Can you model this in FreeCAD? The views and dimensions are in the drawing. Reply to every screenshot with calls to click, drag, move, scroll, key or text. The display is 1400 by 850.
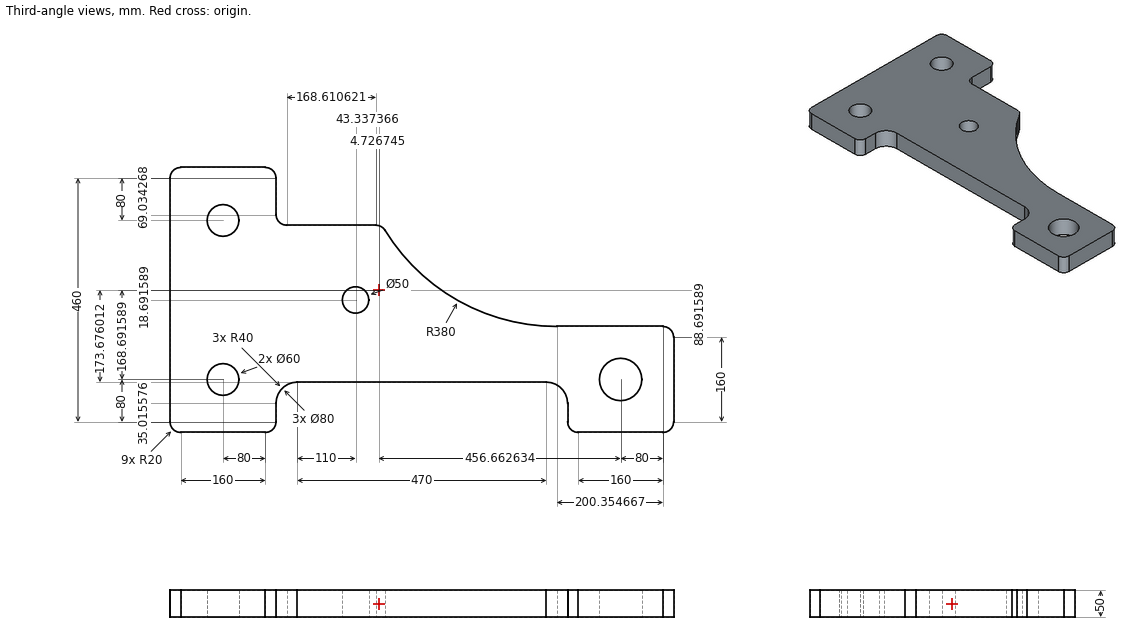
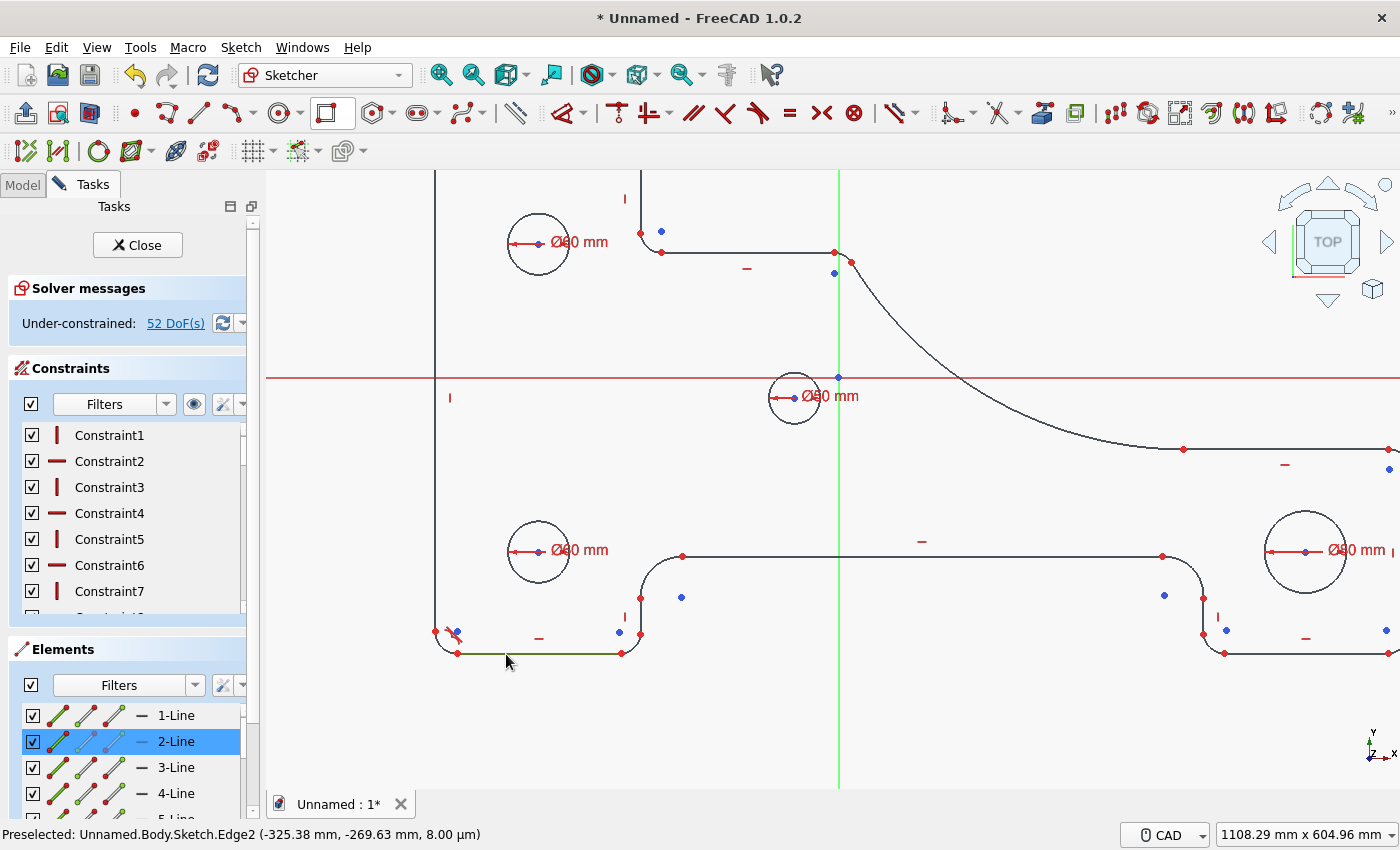
click(634, 648)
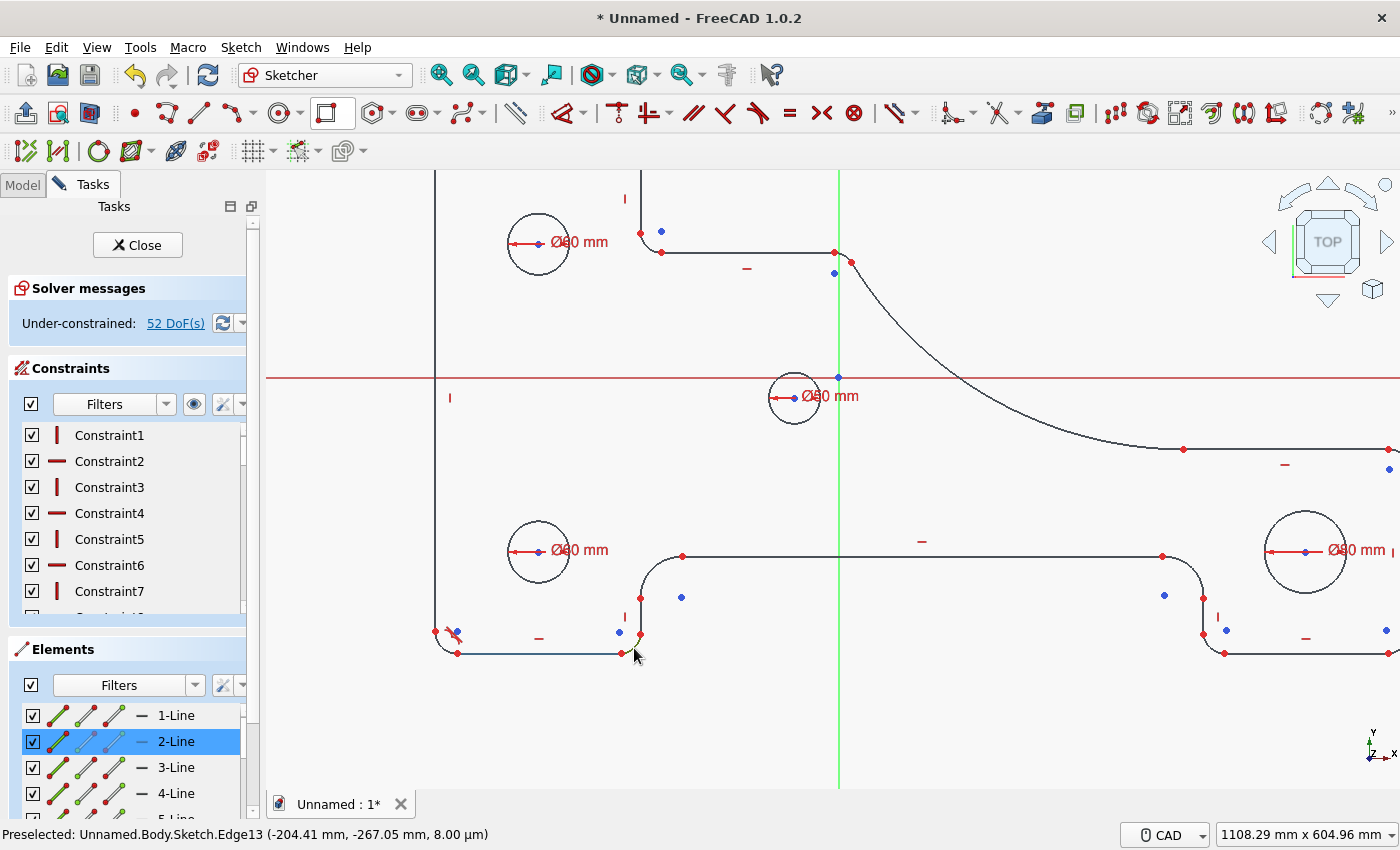
click(758, 114)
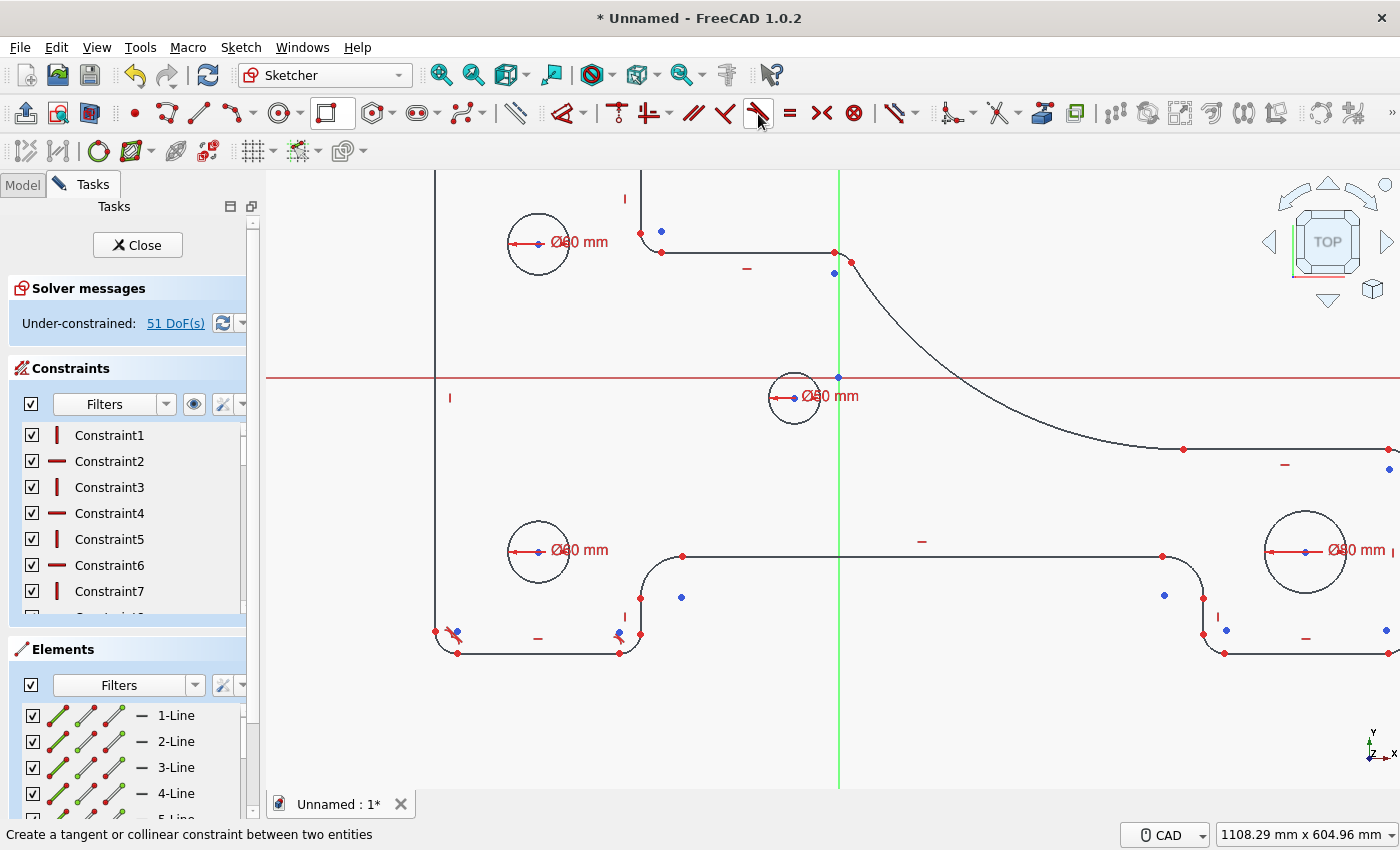
scroll(641, 624, up, 2)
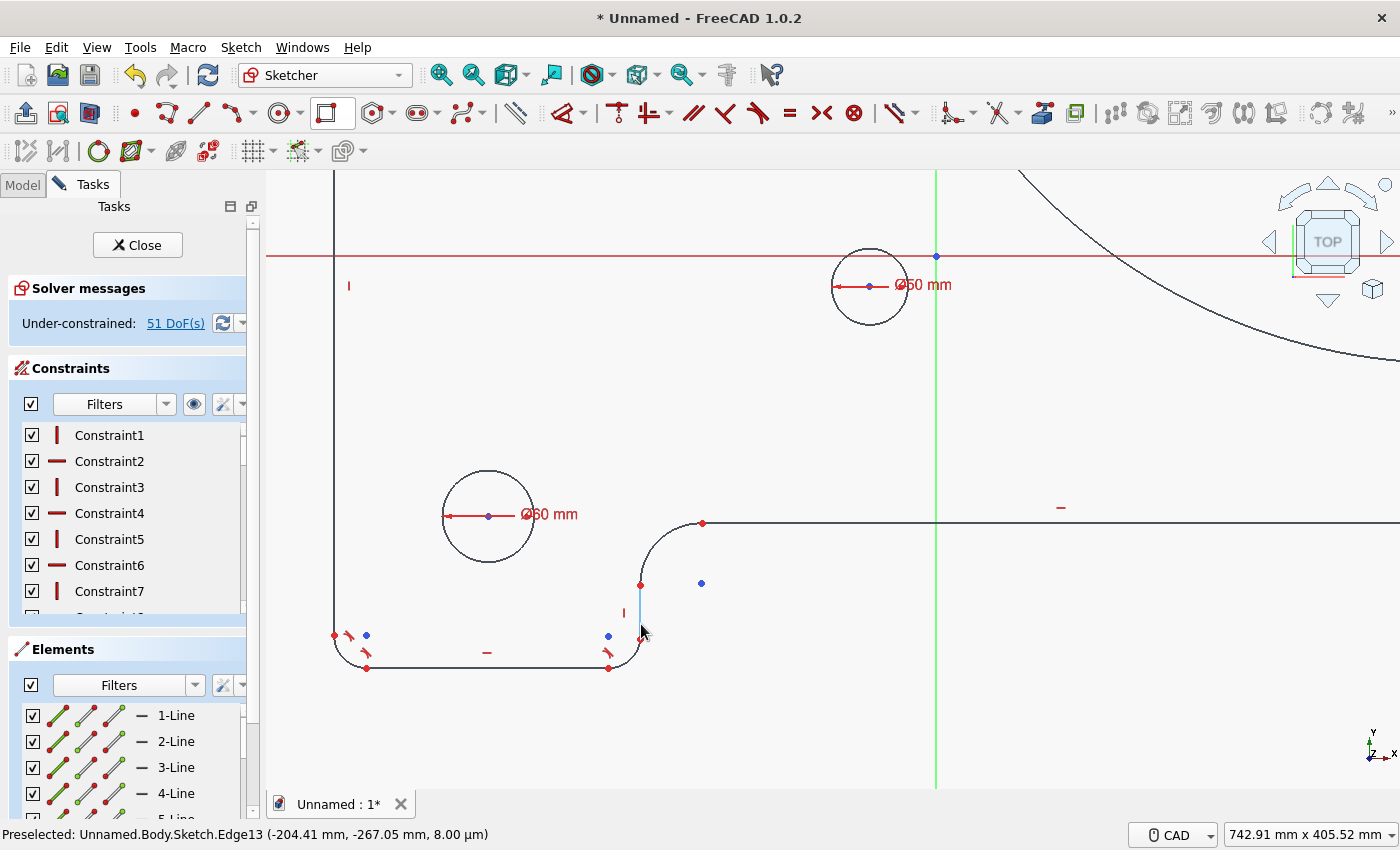
click(640, 623)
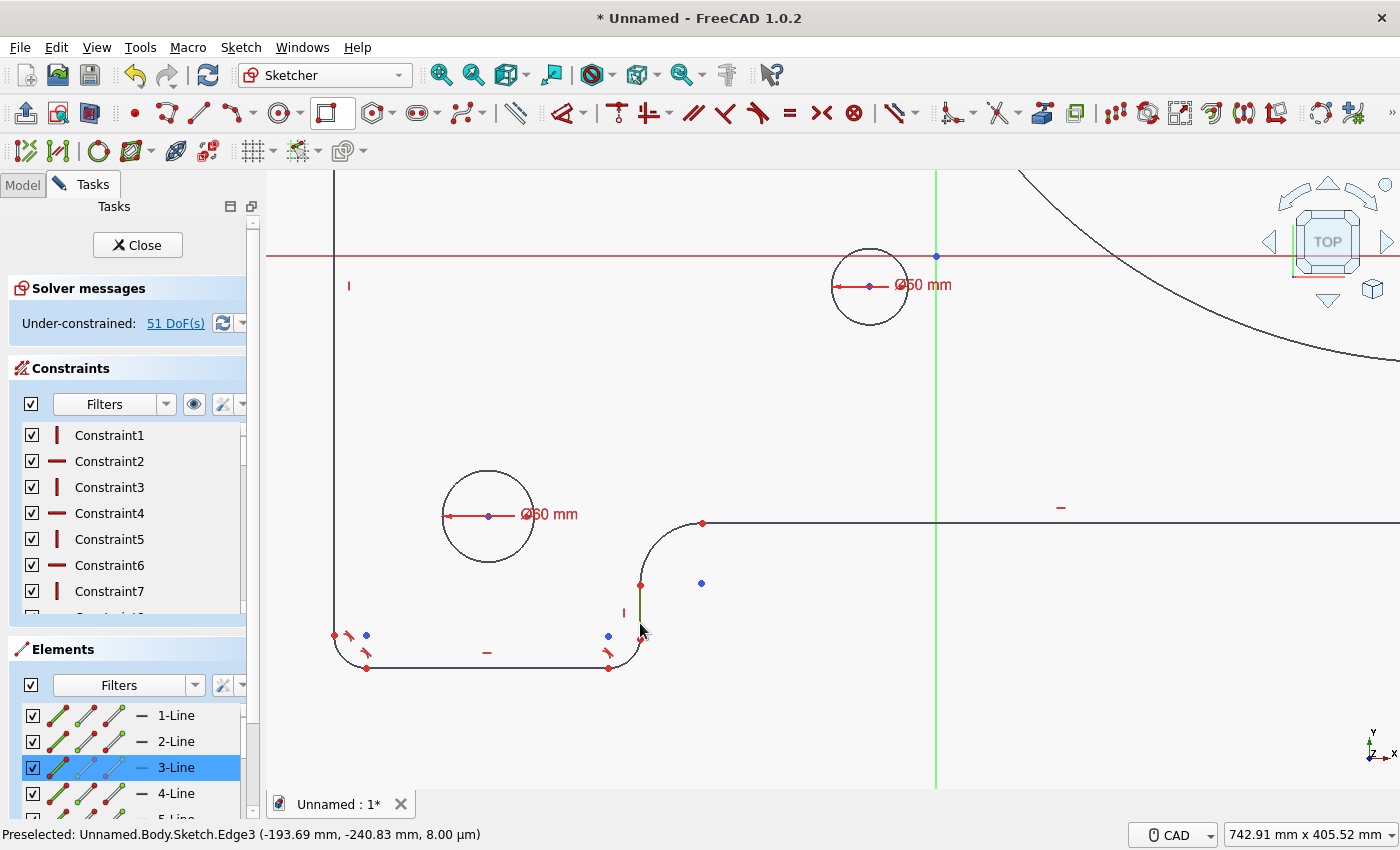
click(622, 665)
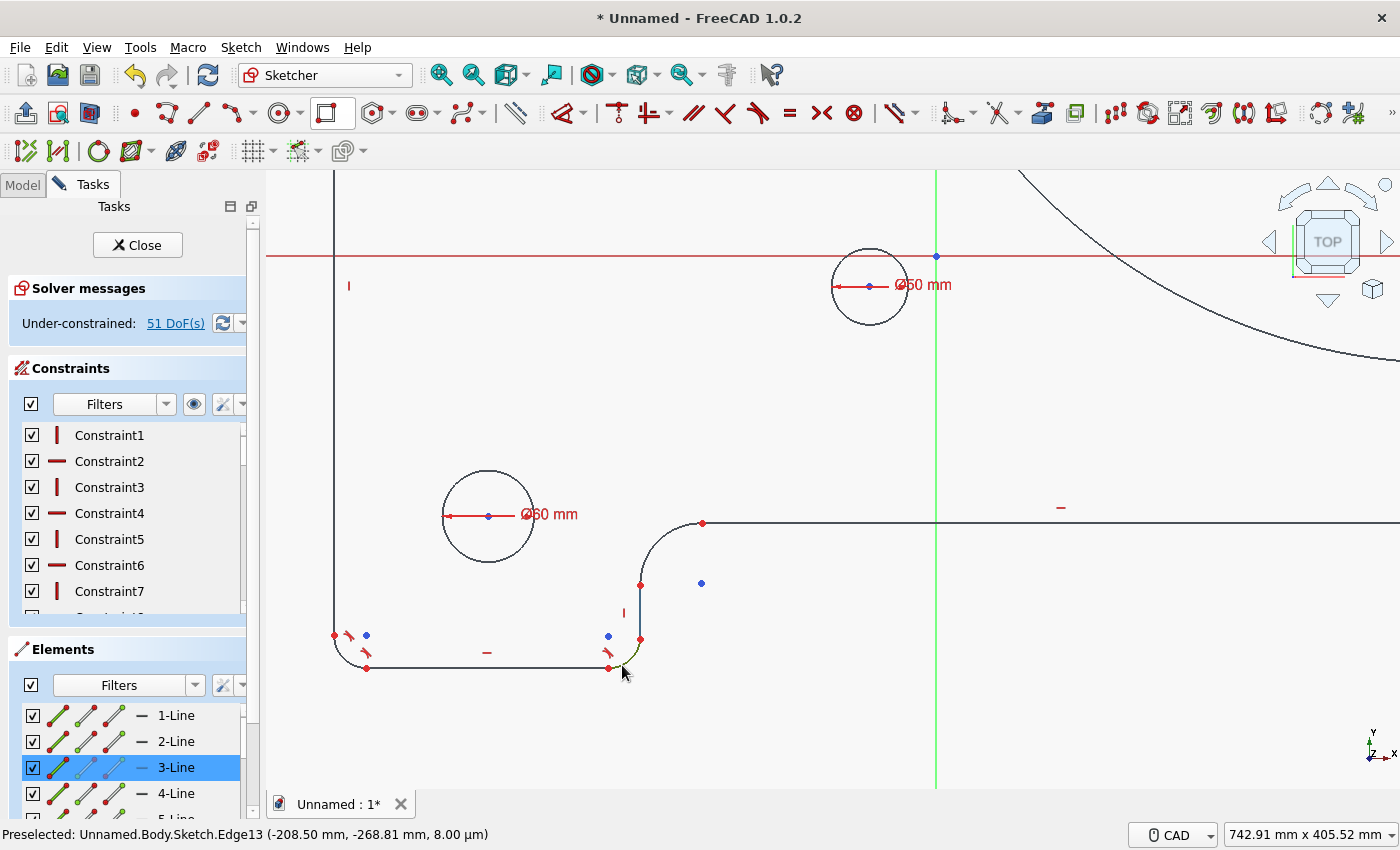
click(758, 114)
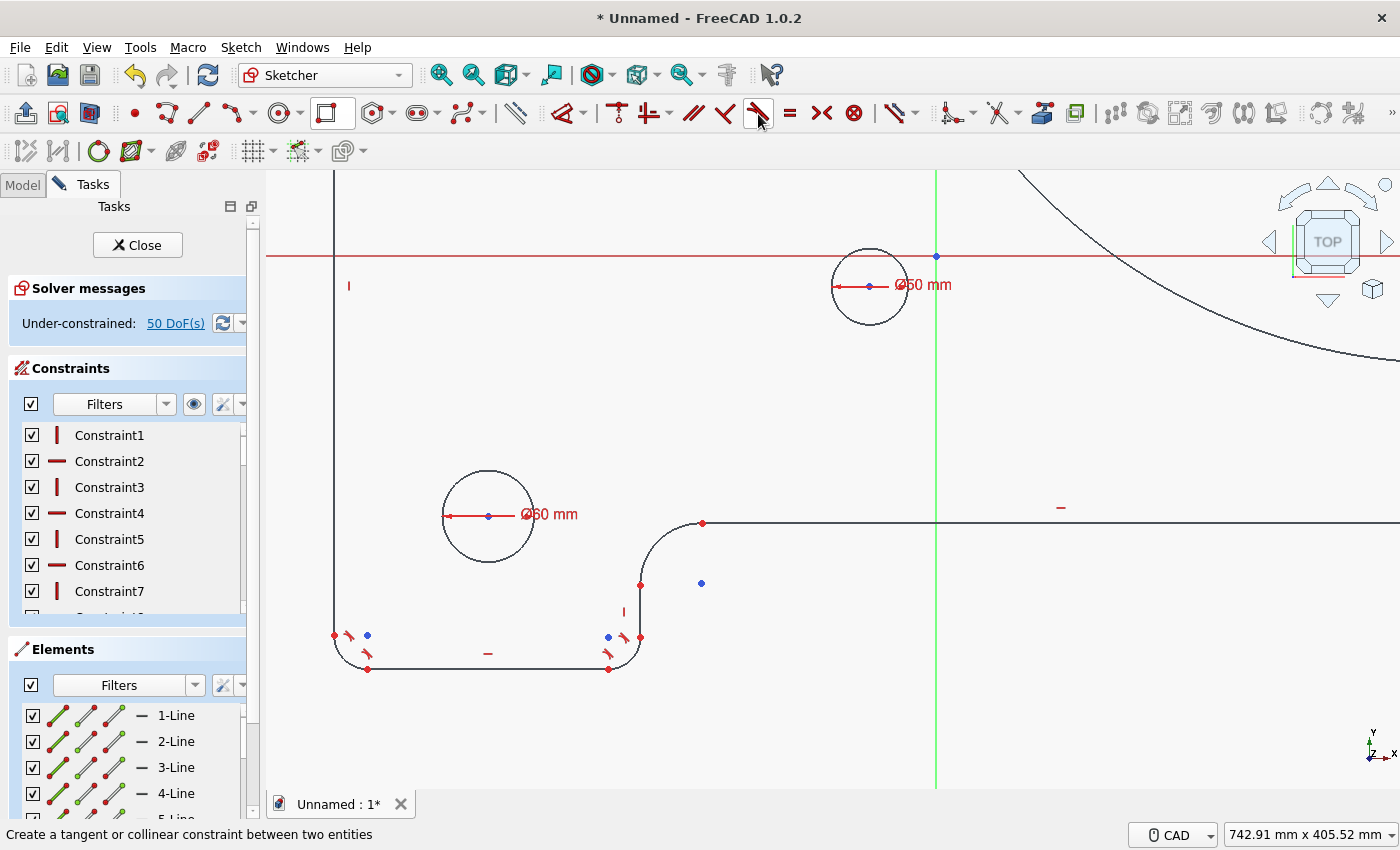
scroll(523, 638, down, 4)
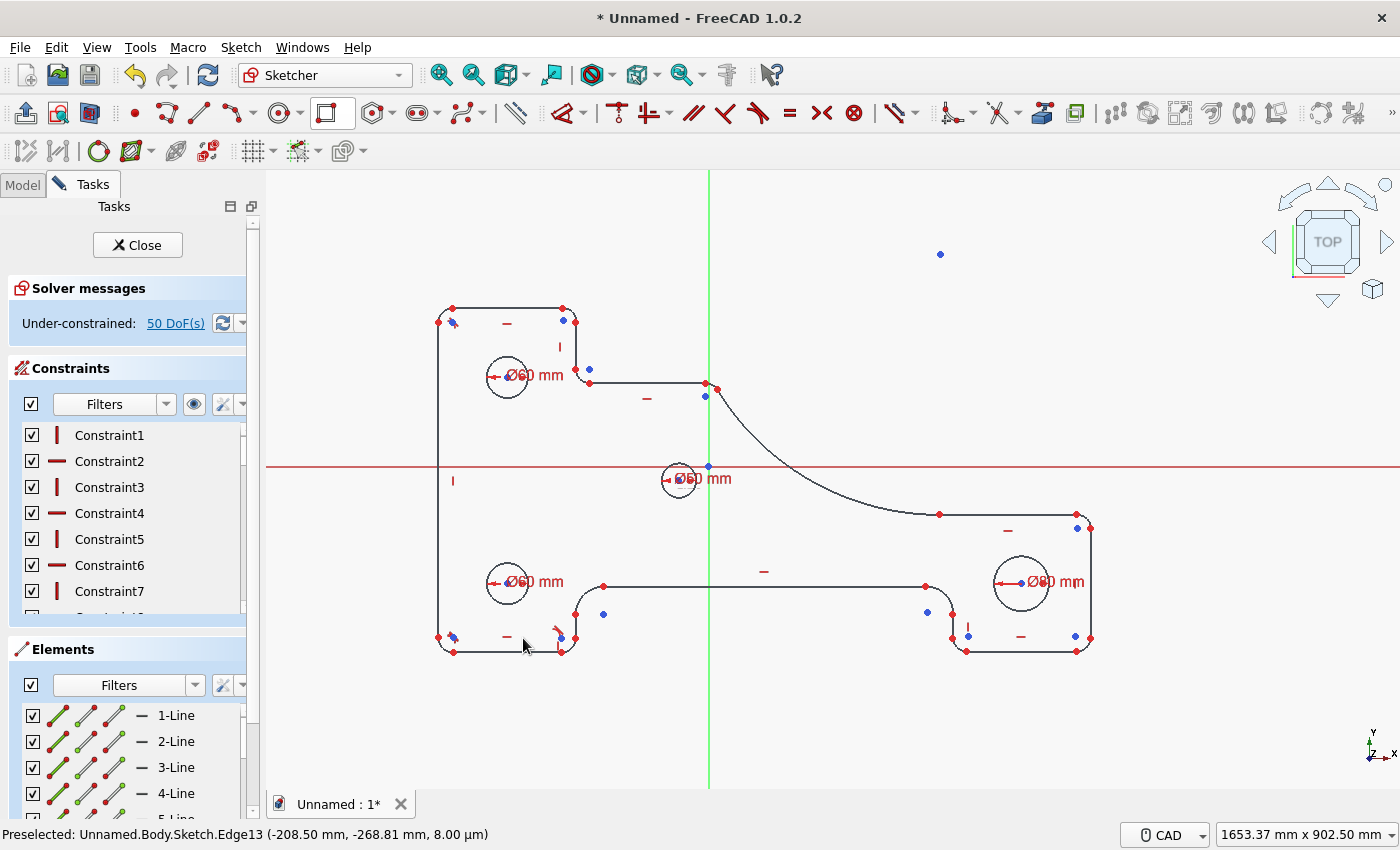
scroll(953, 622, up, 4)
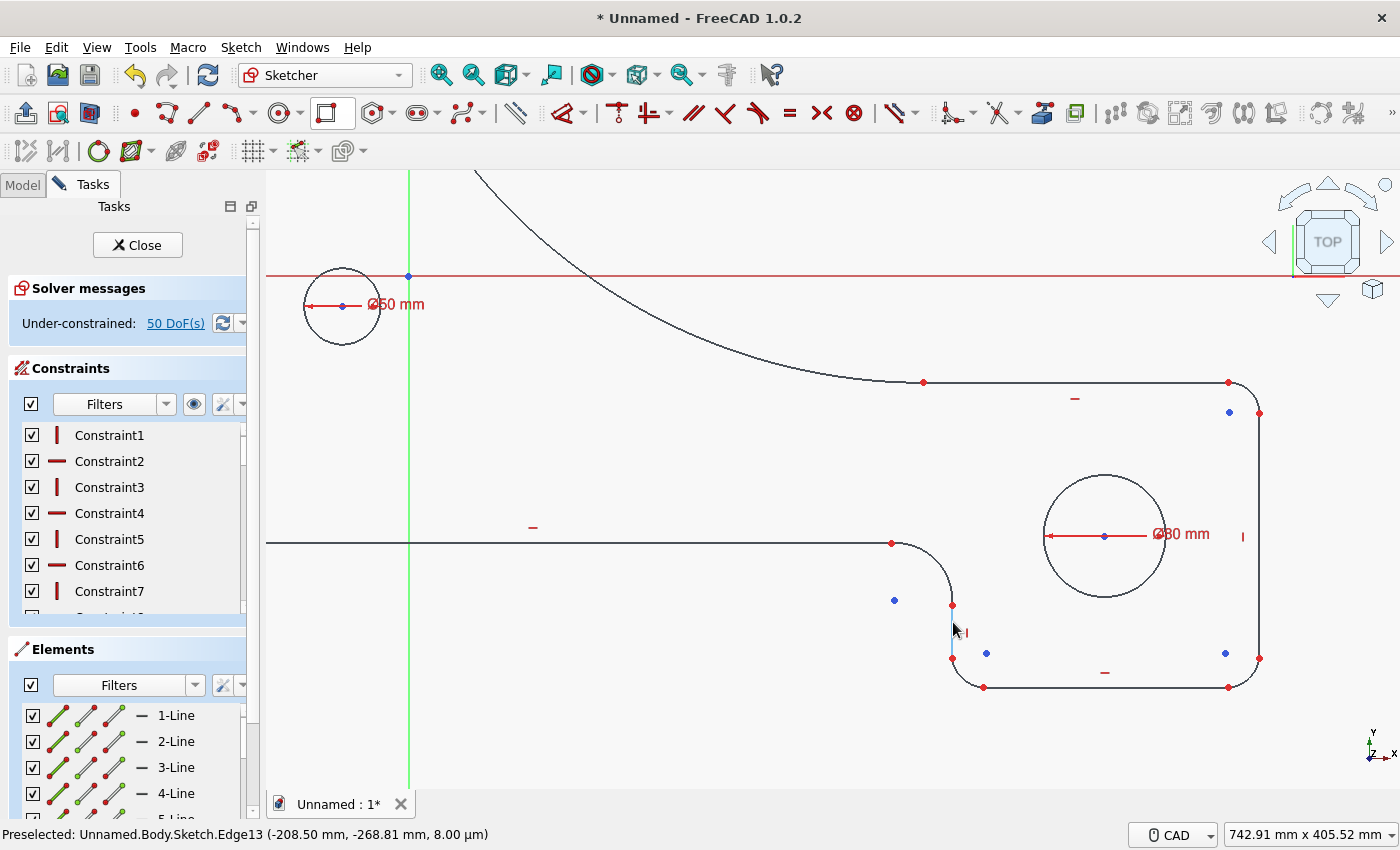
click(952, 621)